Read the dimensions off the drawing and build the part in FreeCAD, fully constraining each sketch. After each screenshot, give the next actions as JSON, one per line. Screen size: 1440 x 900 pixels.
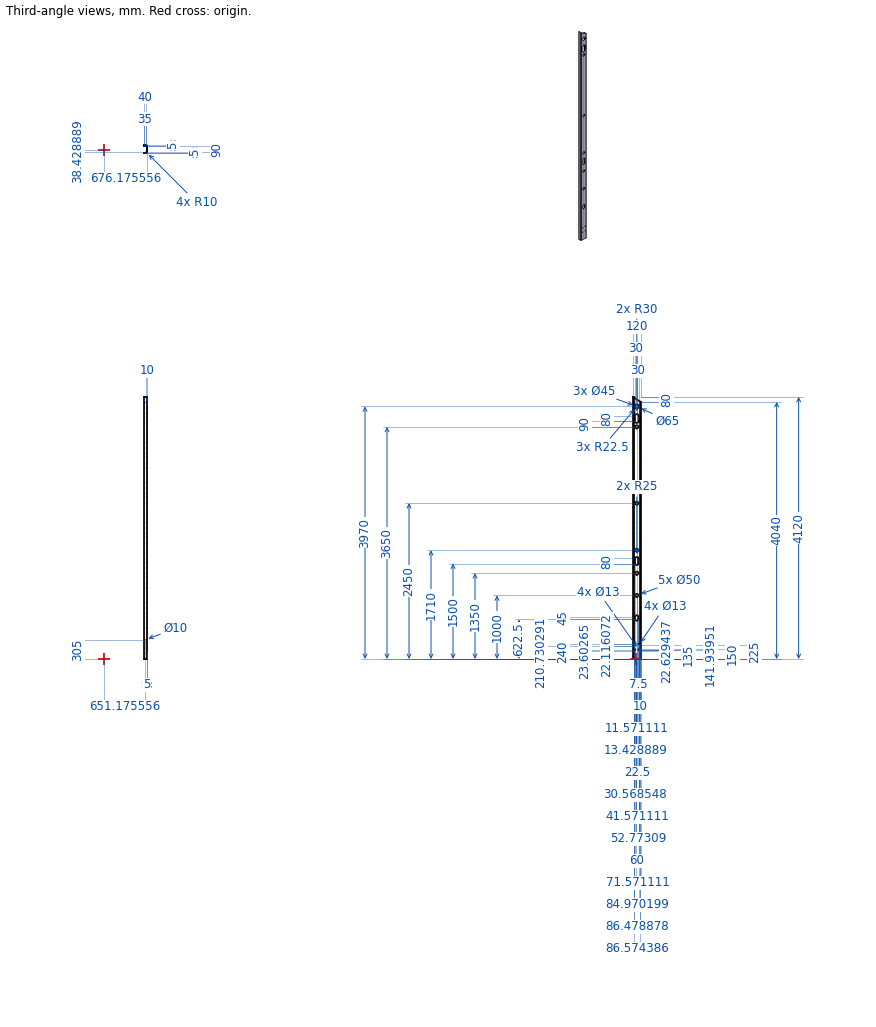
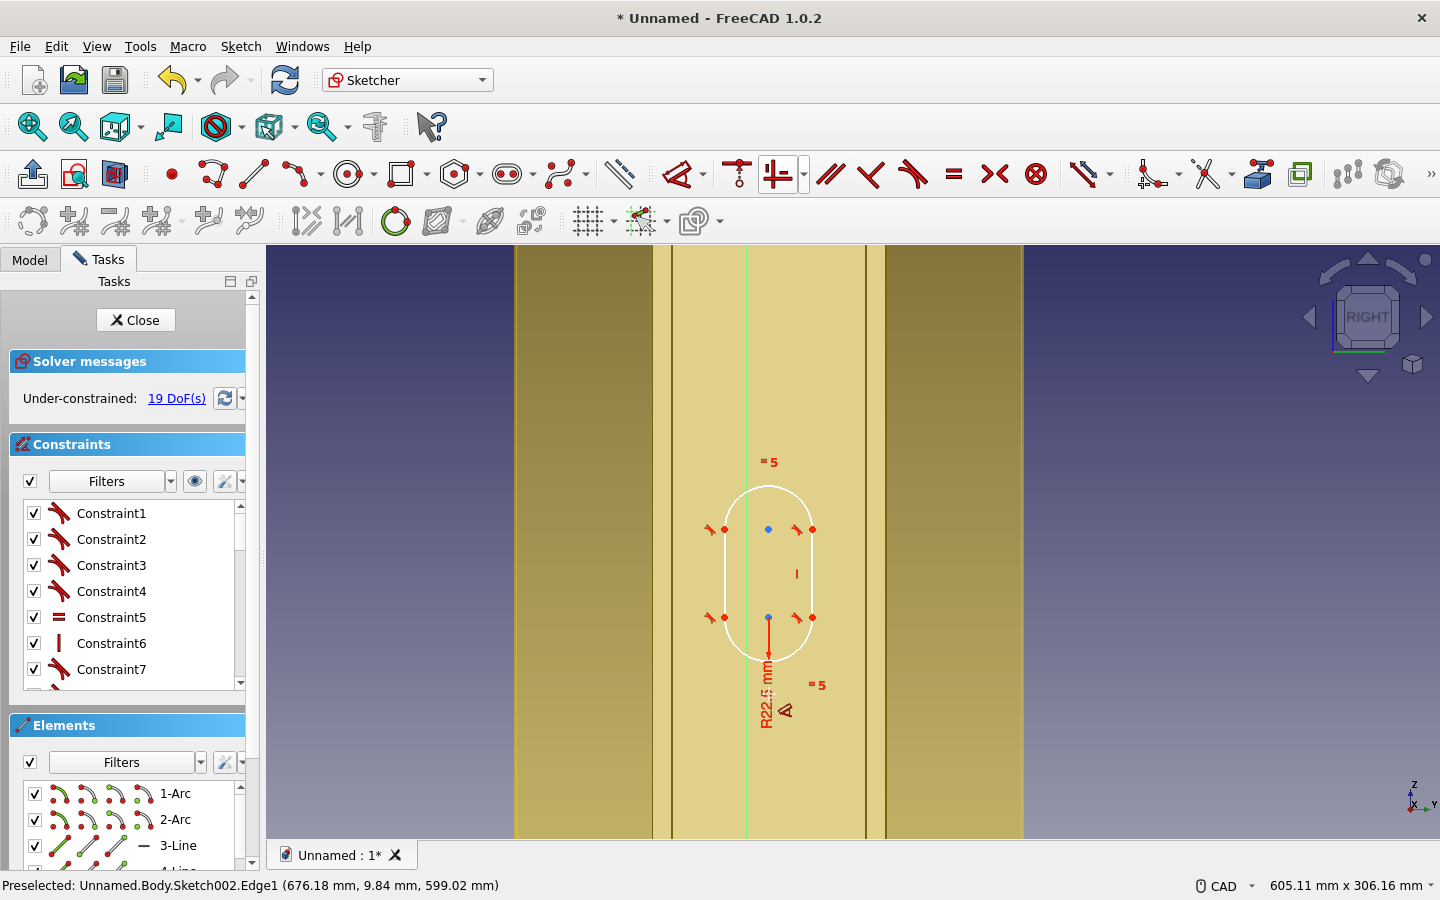
{"action": "scroll", "coordinate": [785, 678], "scroll_direction": "down", "scroll_amount": 15}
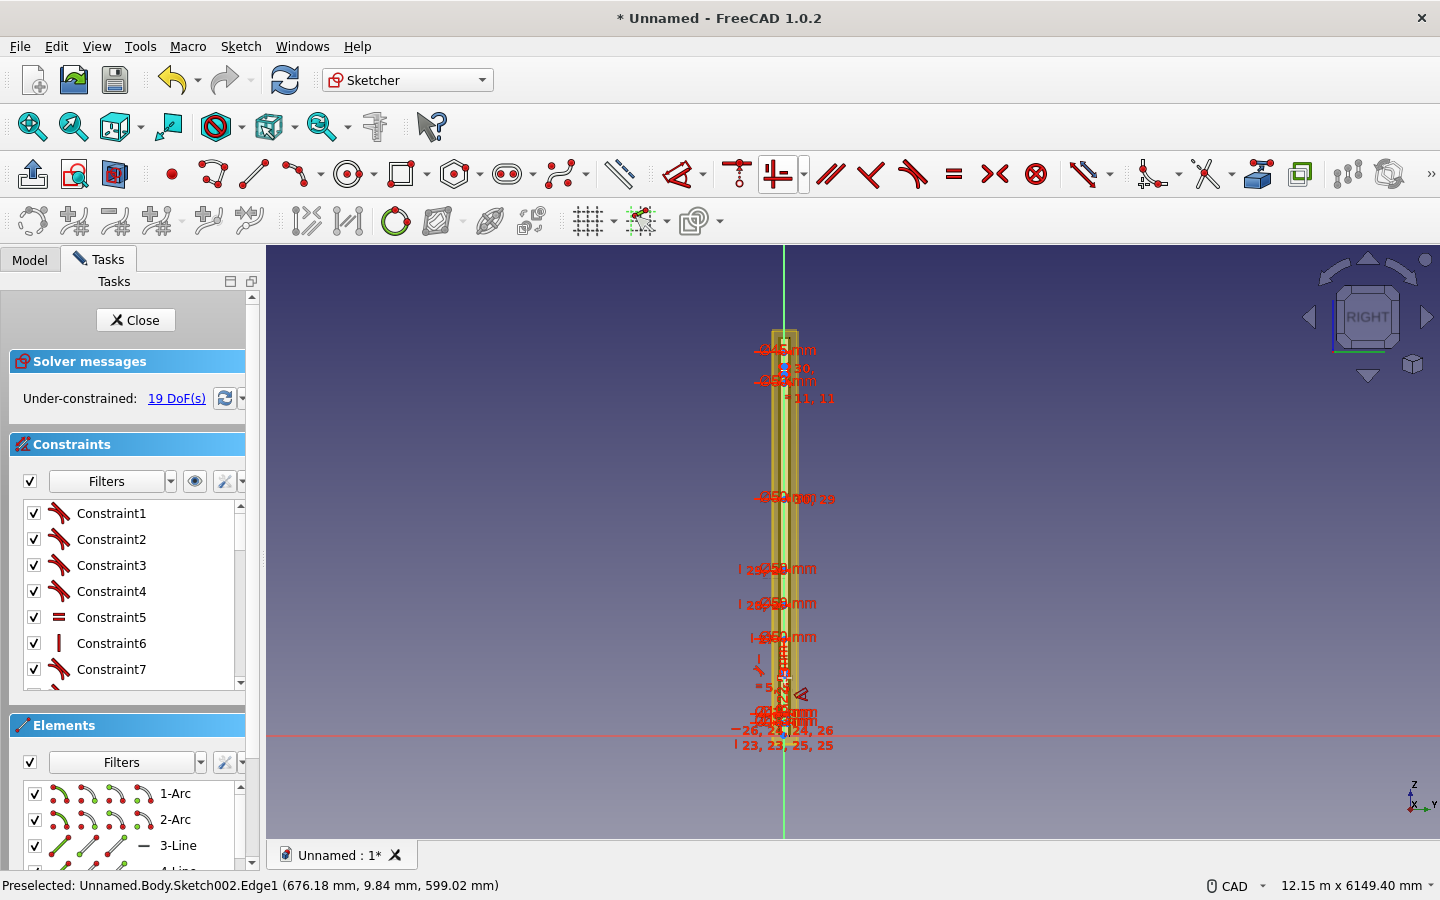
{"action": "scroll", "coordinate": [783, 377], "scroll_direction": "up", "scroll_amount": 14}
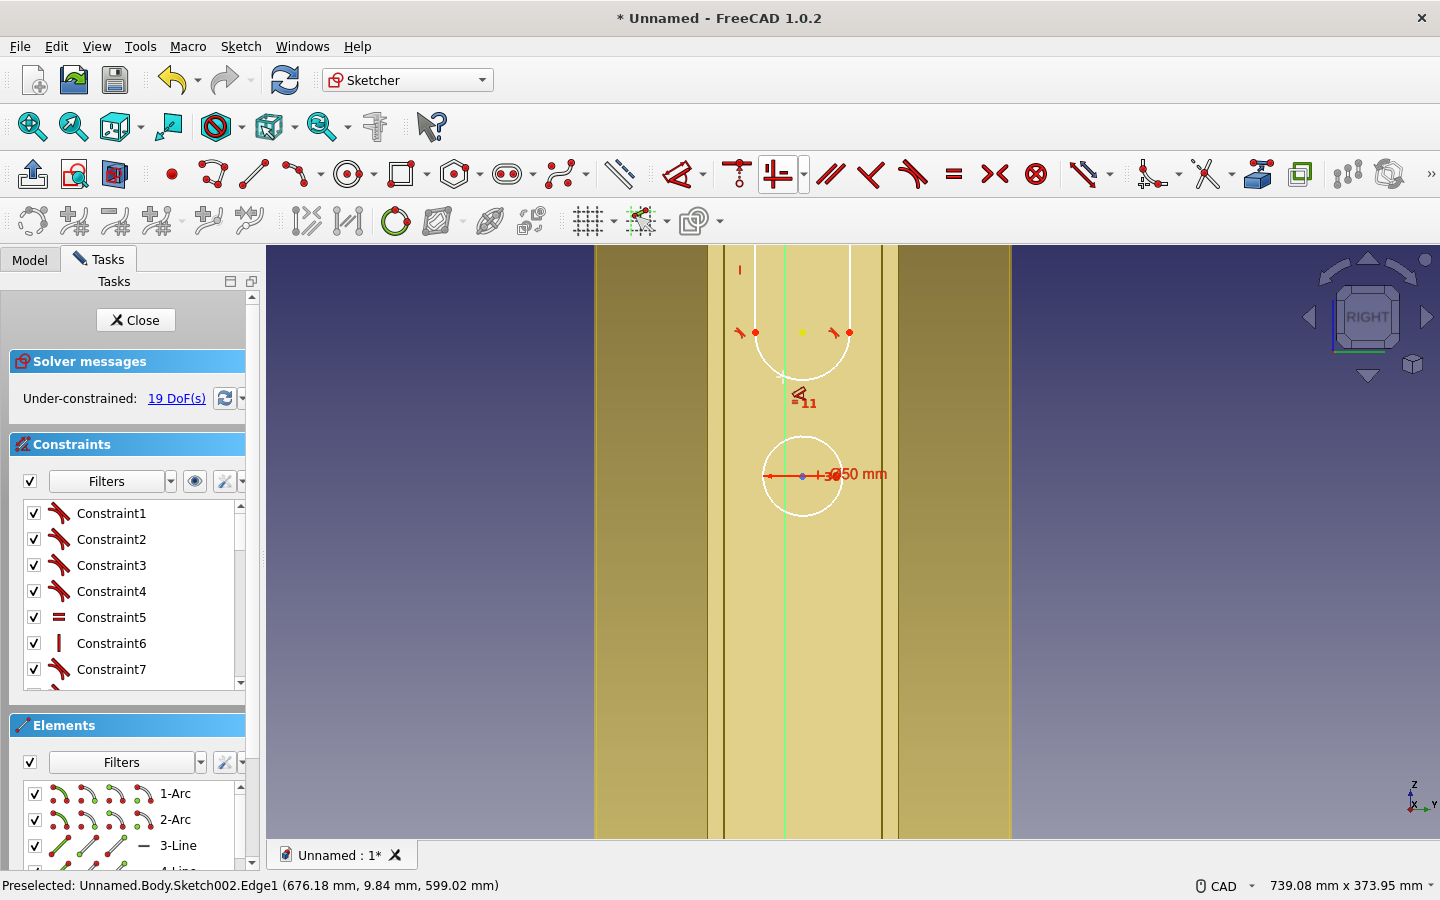
{"action": "left_click", "coordinate": [775, 371]}
{"action": "left_click", "coordinate": [756, 397]}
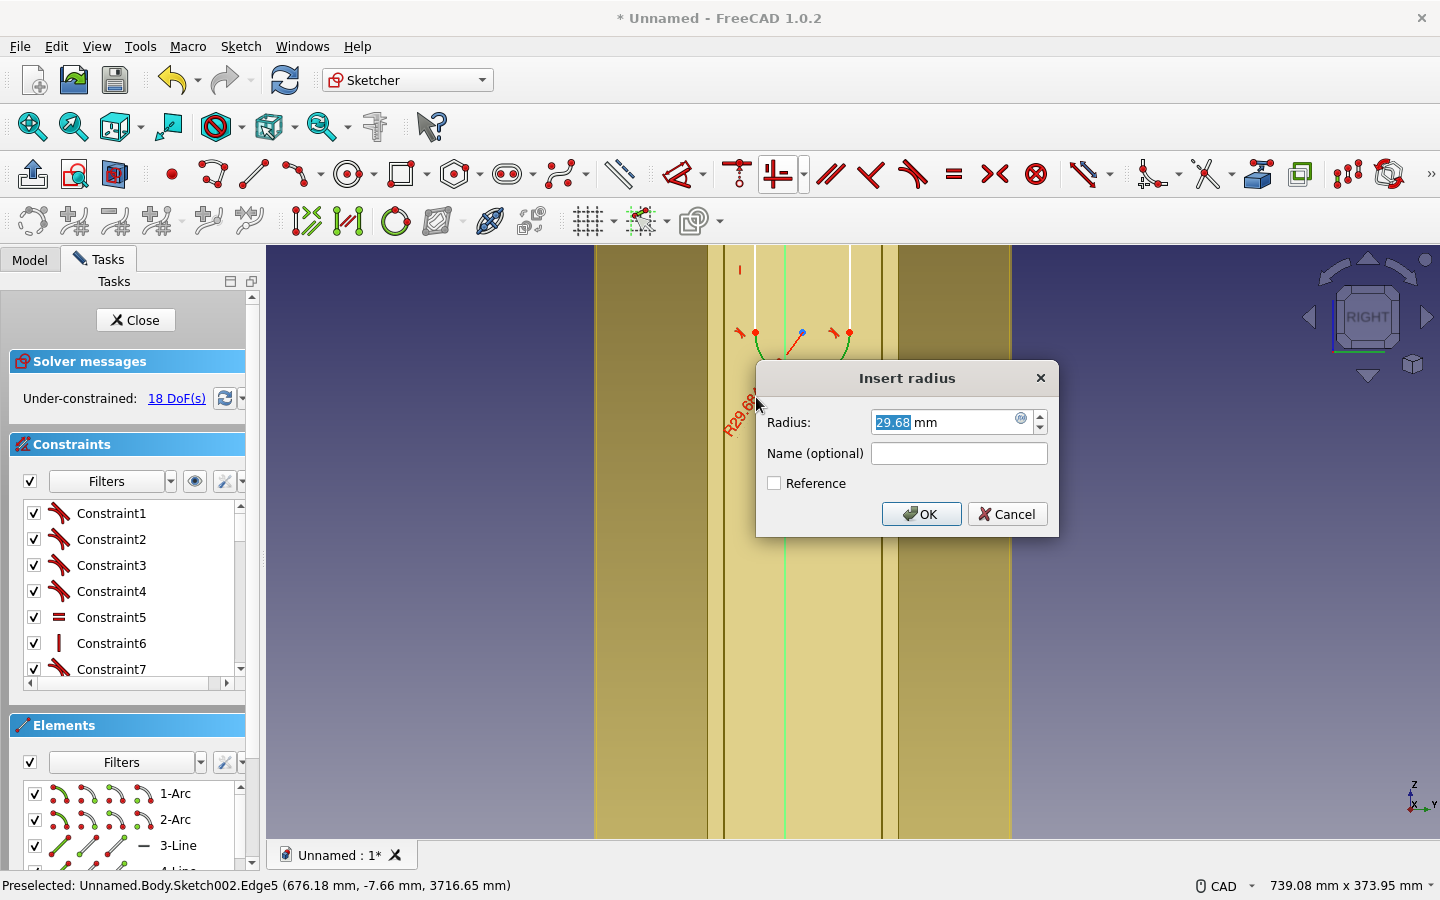
{"action": "type", "text": "30"}
{"action": "key", "text": "Return"}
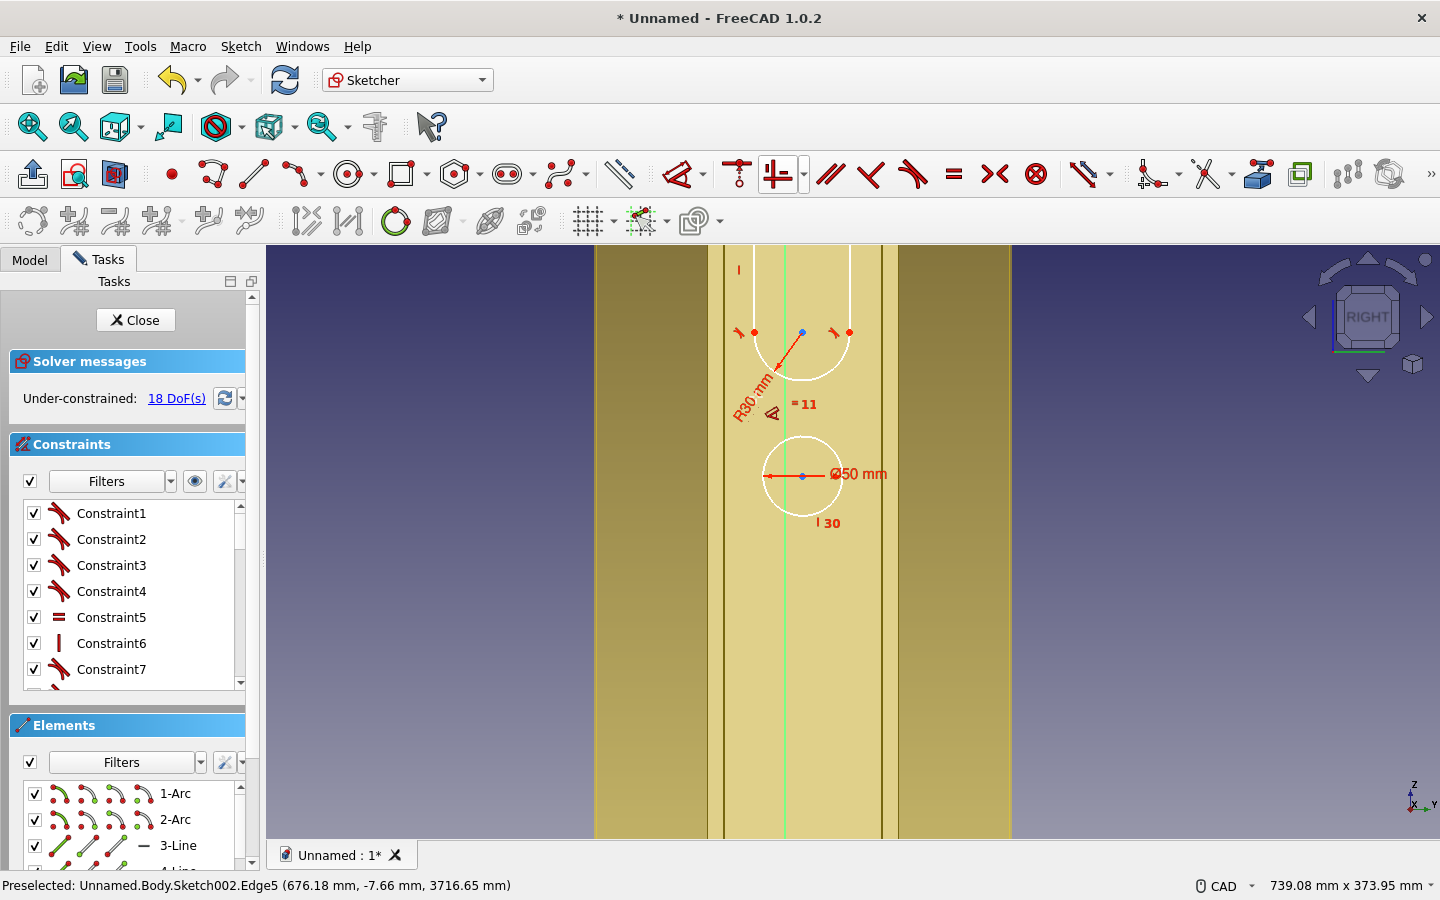
{"action": "scroll", "coordinate": [783, 376], "scroll_direction": "down", "scroll_amount": 14}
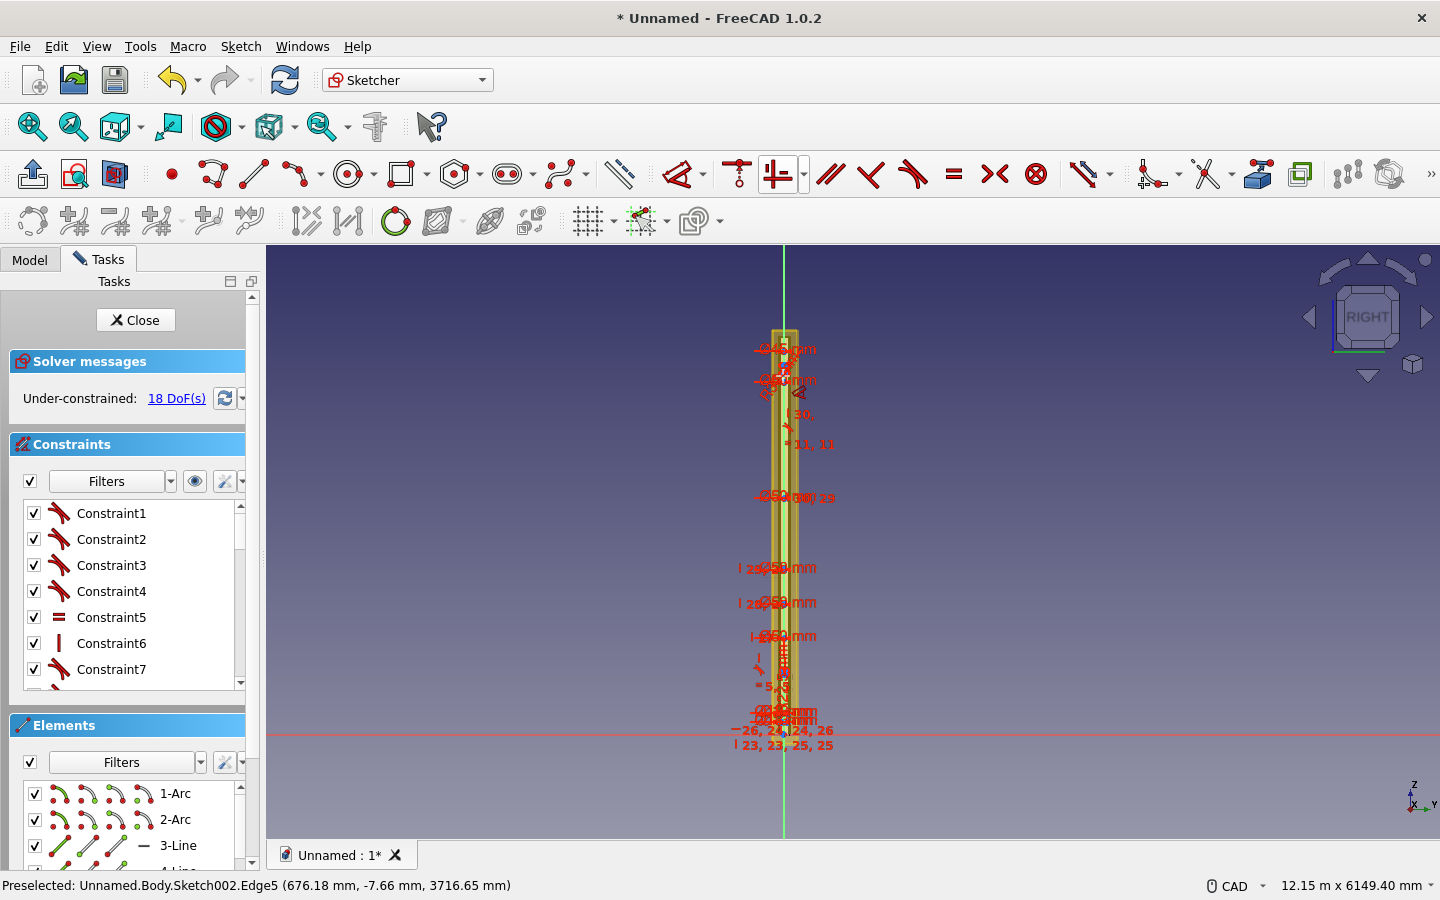
{"action": "scroll", "coordinate": [782, 673], "scroll_direction": "up", "scroll_amount": 13}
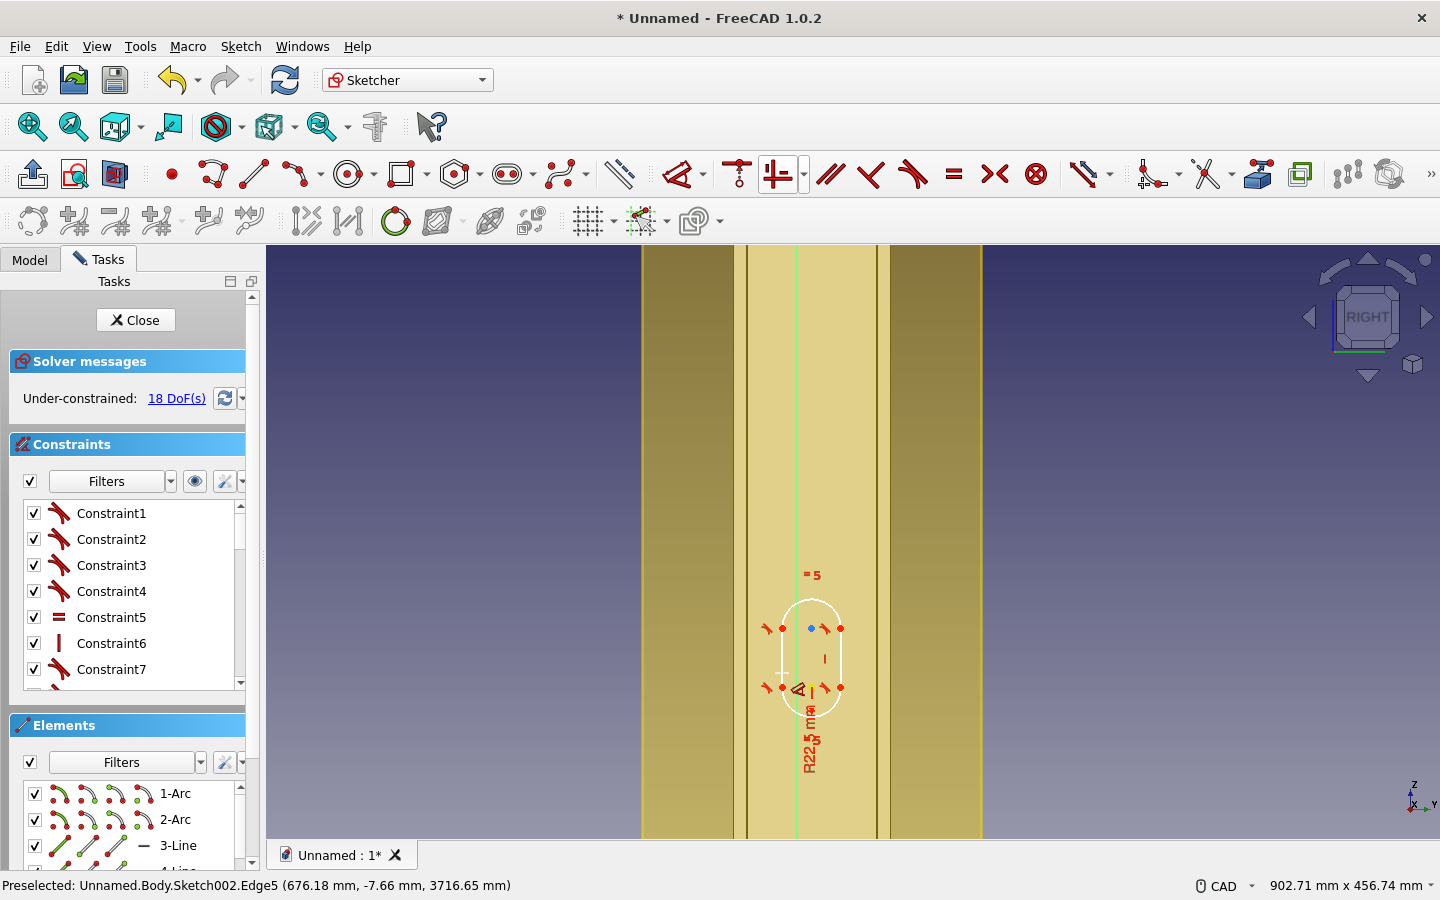
{"action": "left_click", "coordinate": [782, 670]}
{"action": "left_click", "coordinate": [748, 658]}